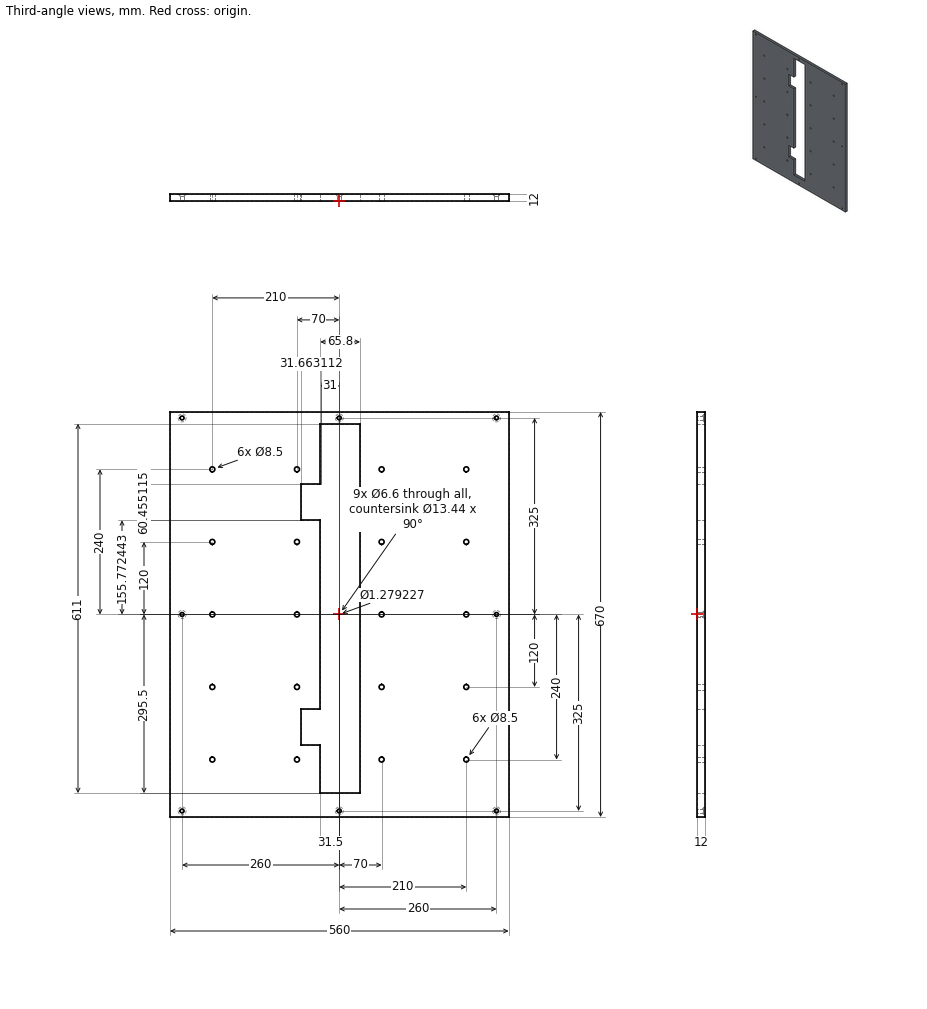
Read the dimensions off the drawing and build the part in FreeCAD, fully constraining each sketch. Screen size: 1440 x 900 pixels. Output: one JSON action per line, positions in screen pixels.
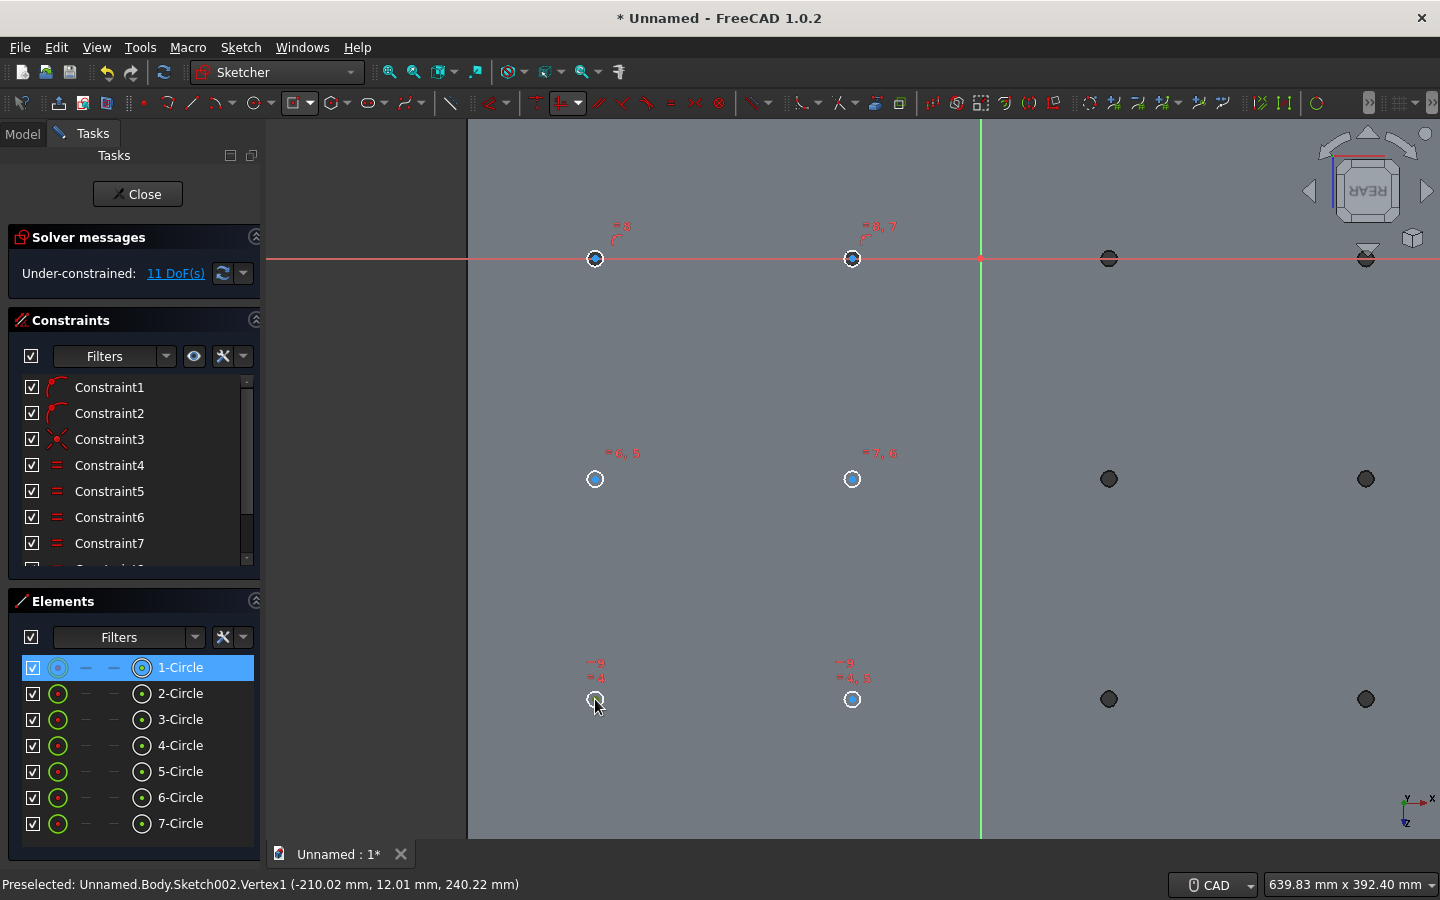
{"action": "left_click", "coordinate": [595, 479]}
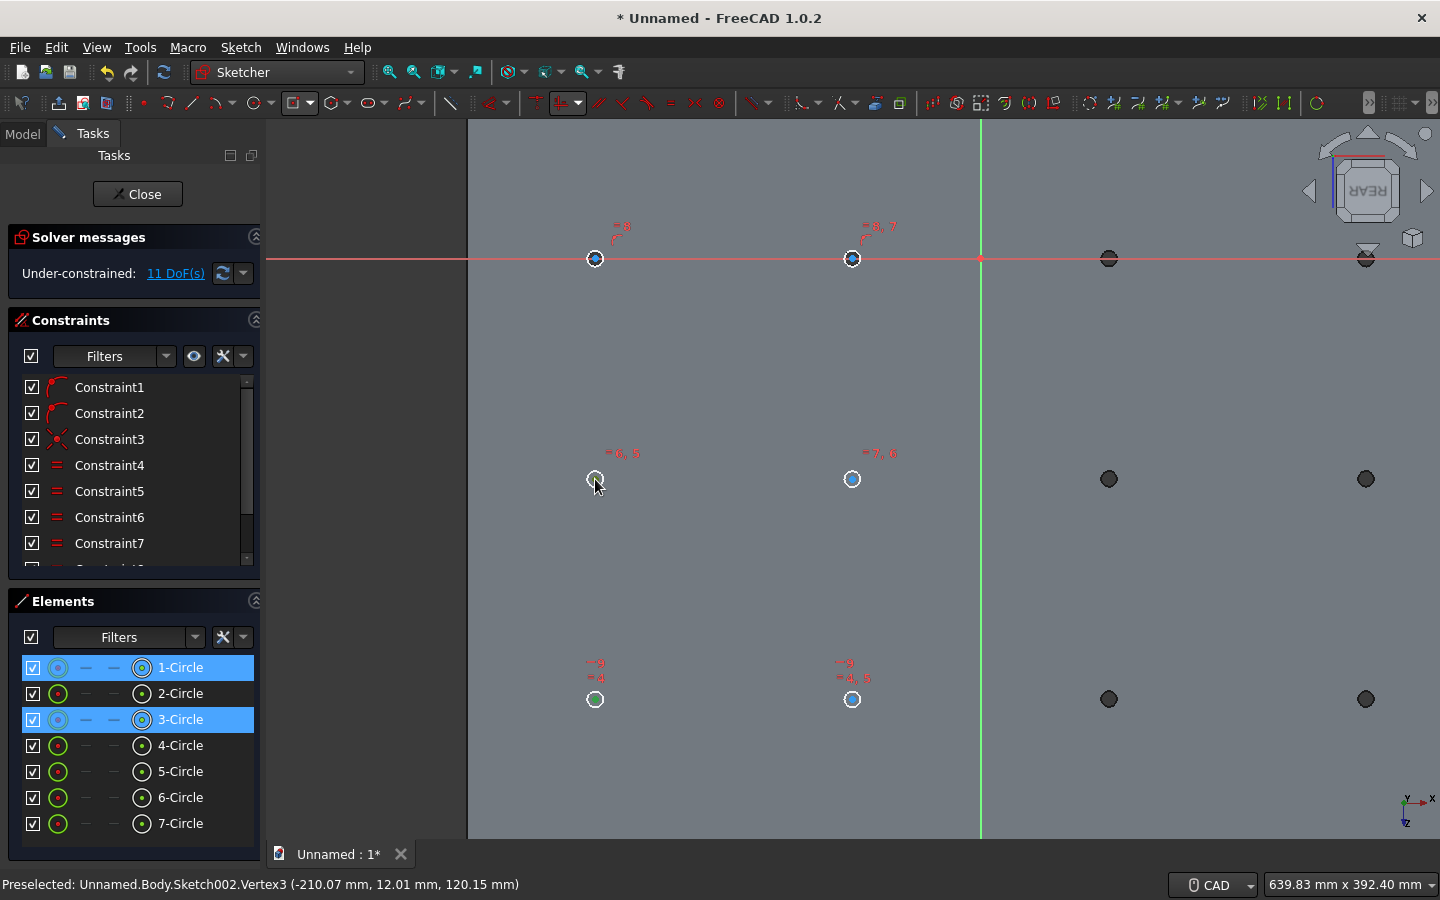
{"action": "key", "text": "v"}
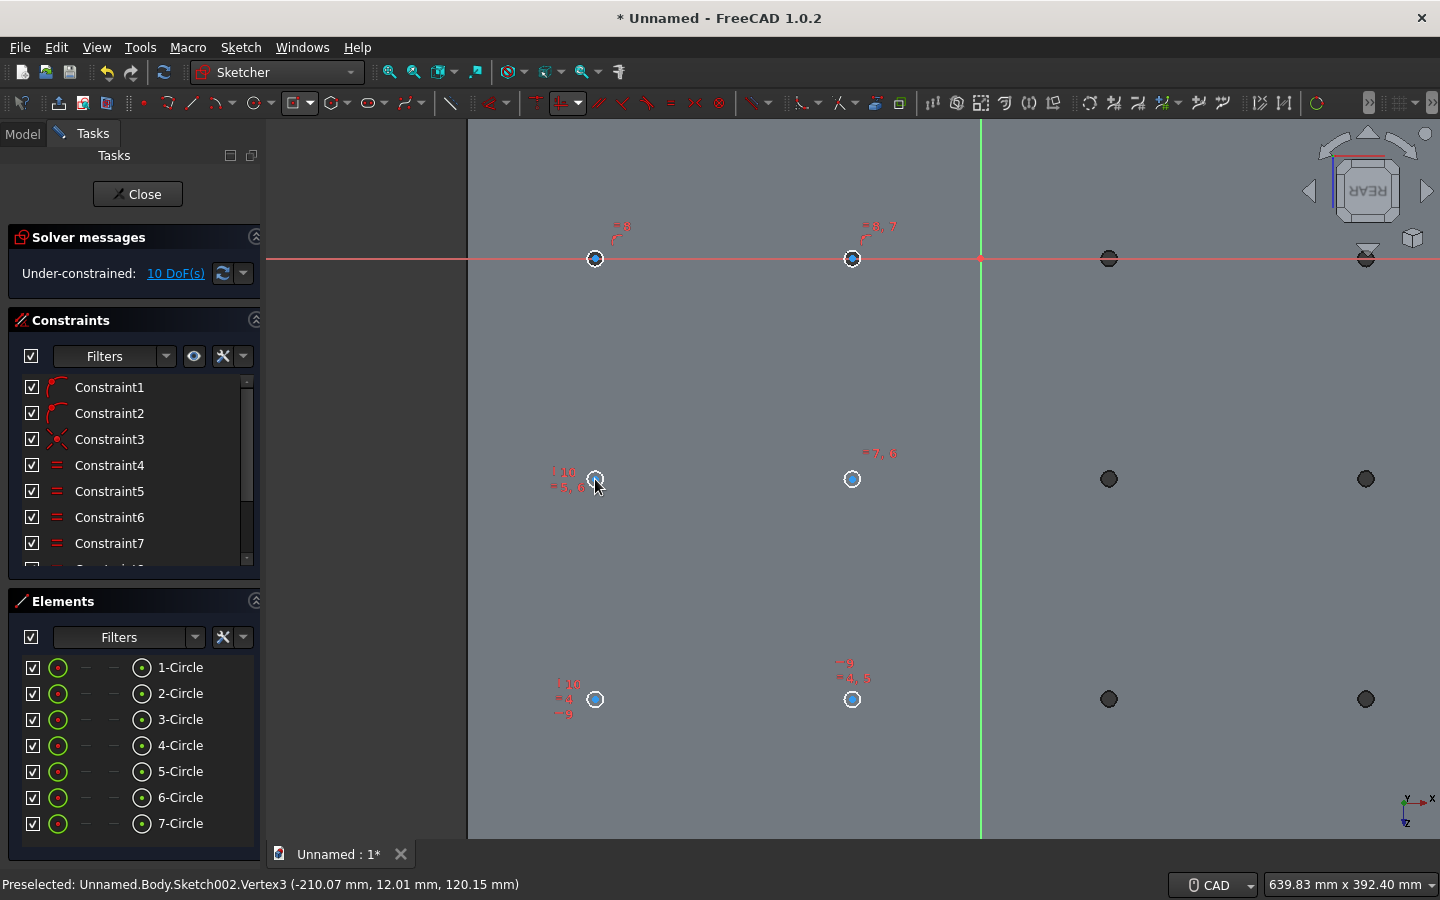
{"action": "left_click", "coordinate": [852, 699]}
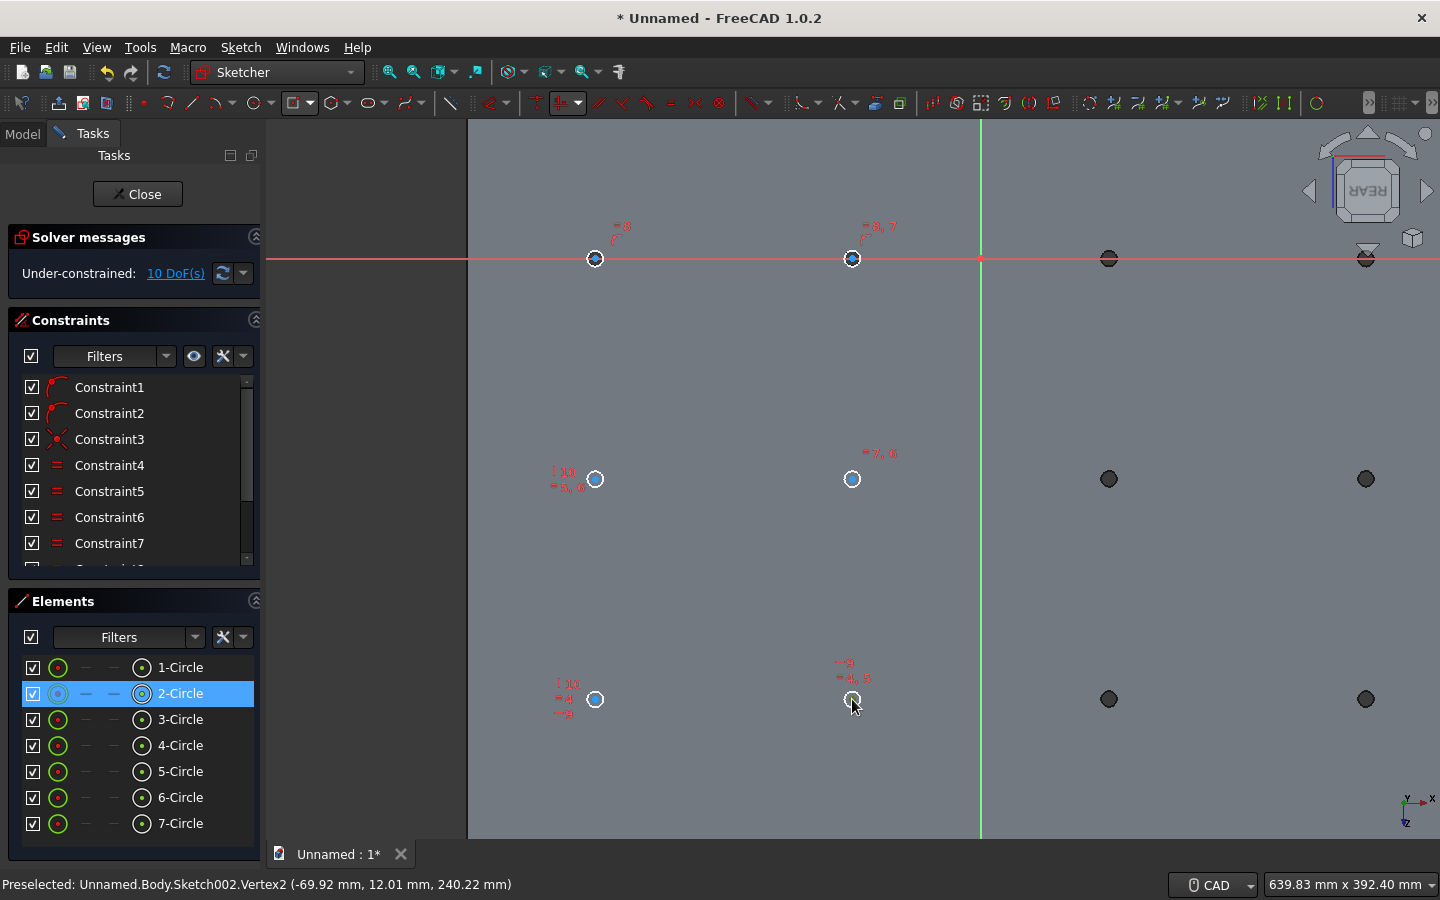
{"action": "left_click", "coordinate": [852, 479]}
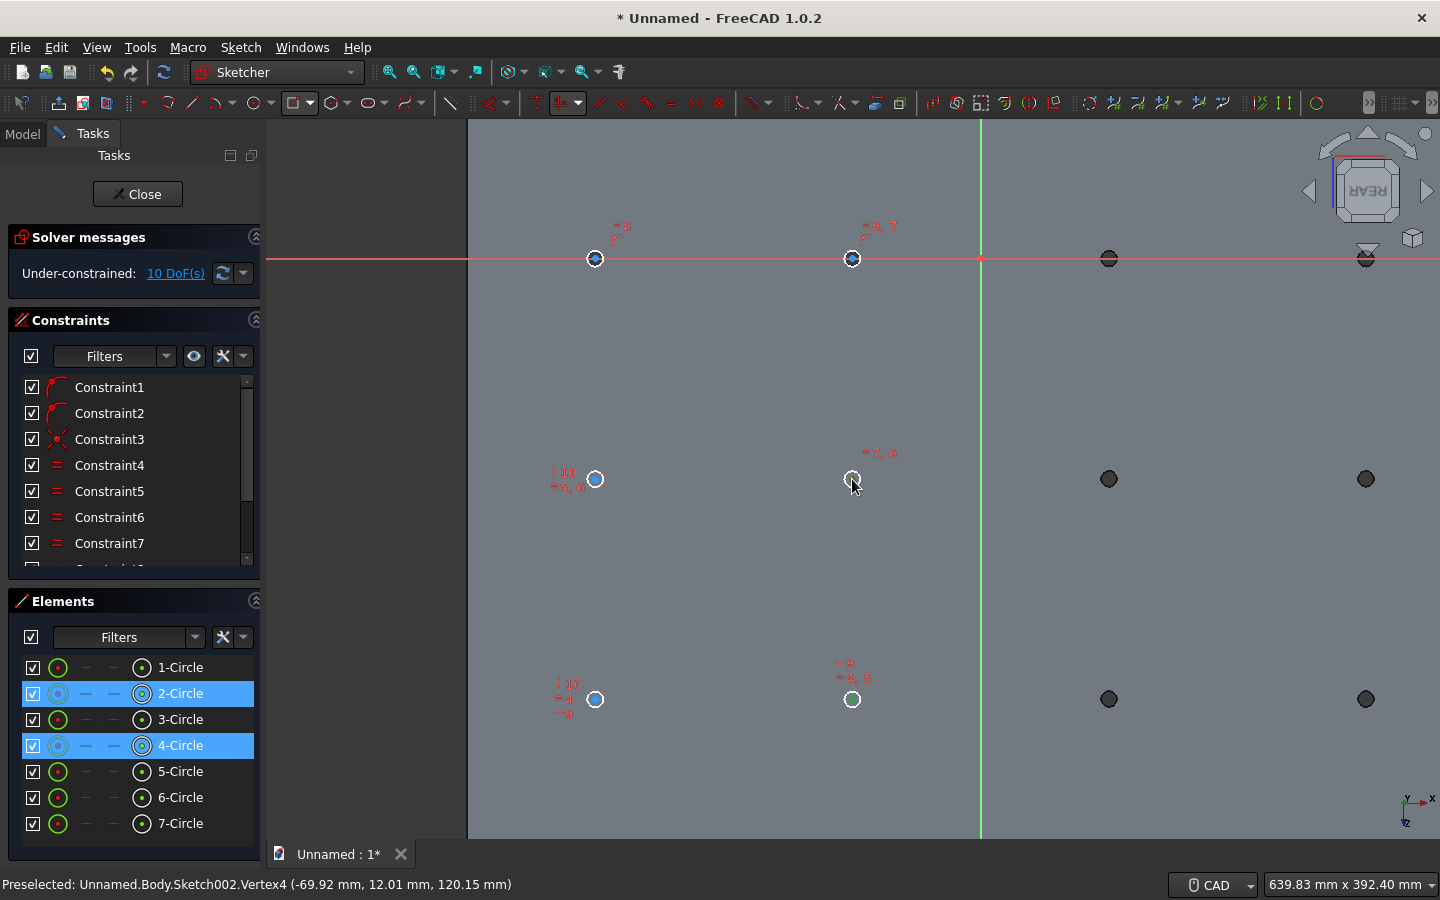
{"action": "left_click", "coordinate": [580, 104]}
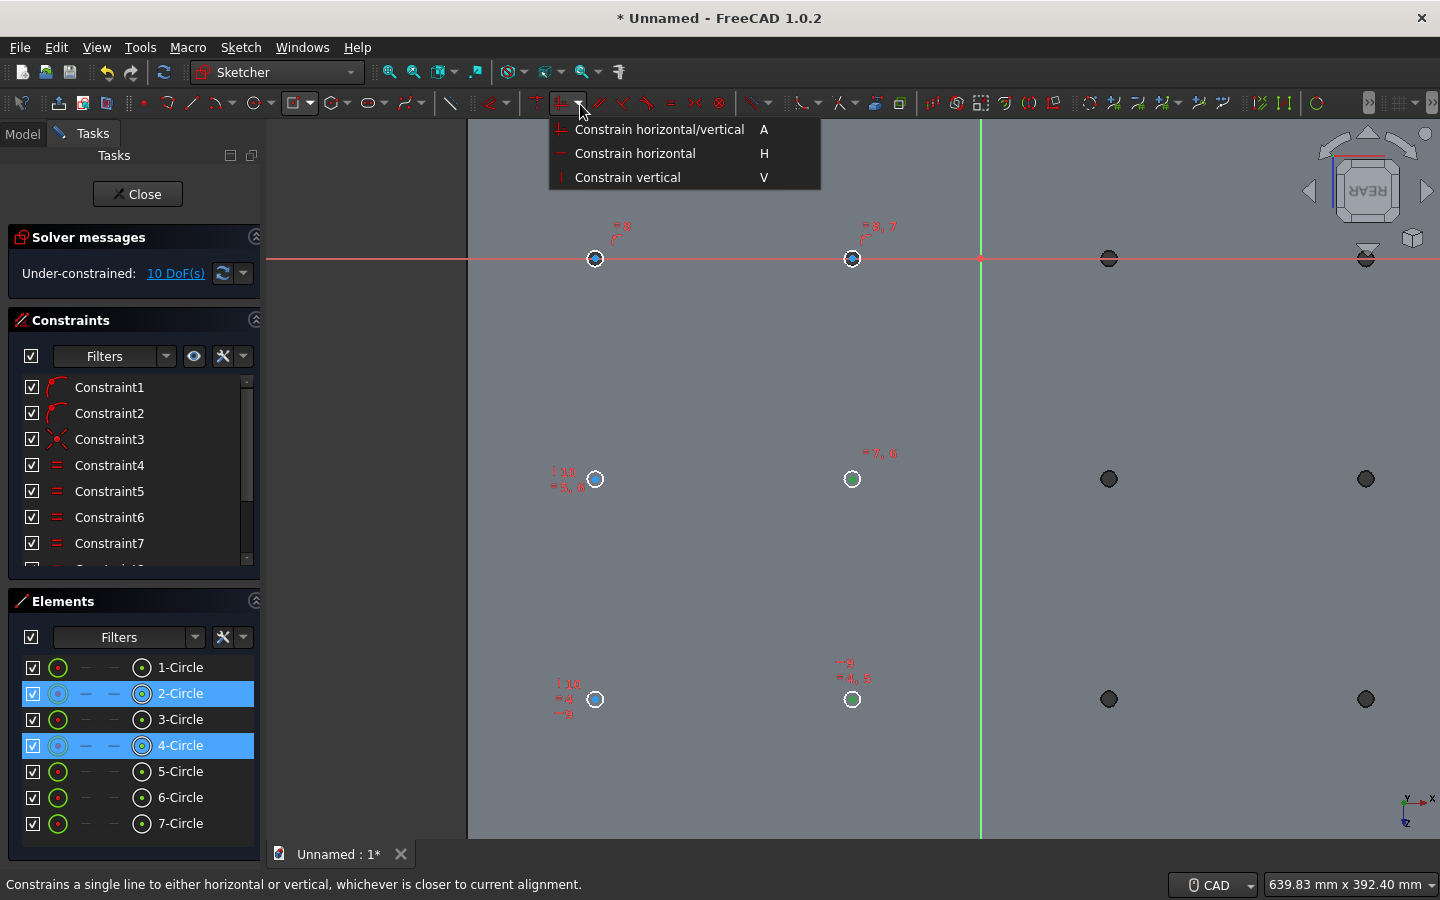
{"action": "left_click", "coordinate": [685, 177]}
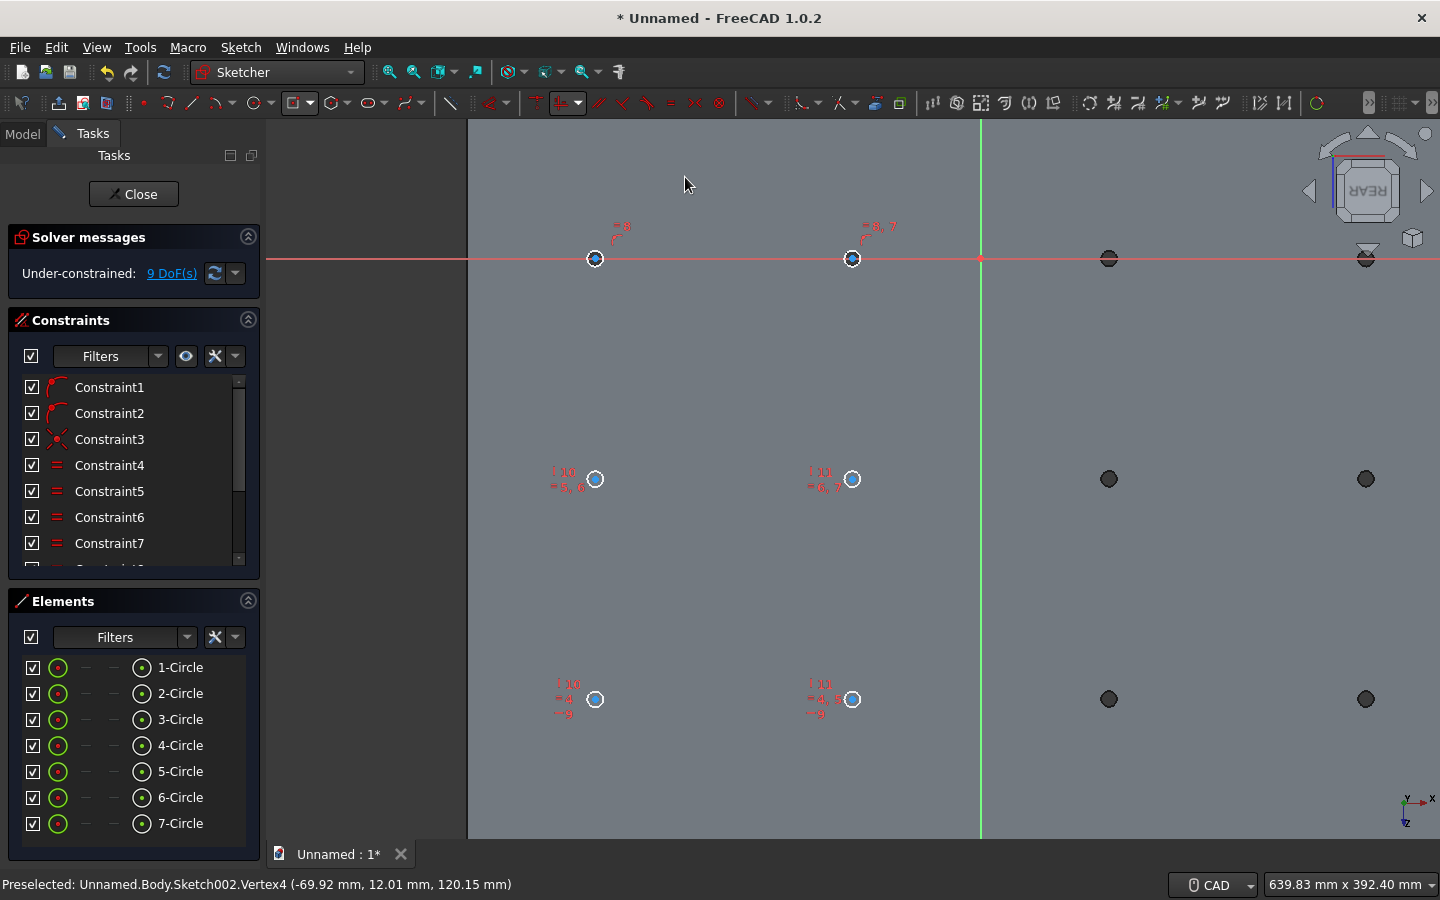
{"action": "left_click", "coordinate": [595, 479]}